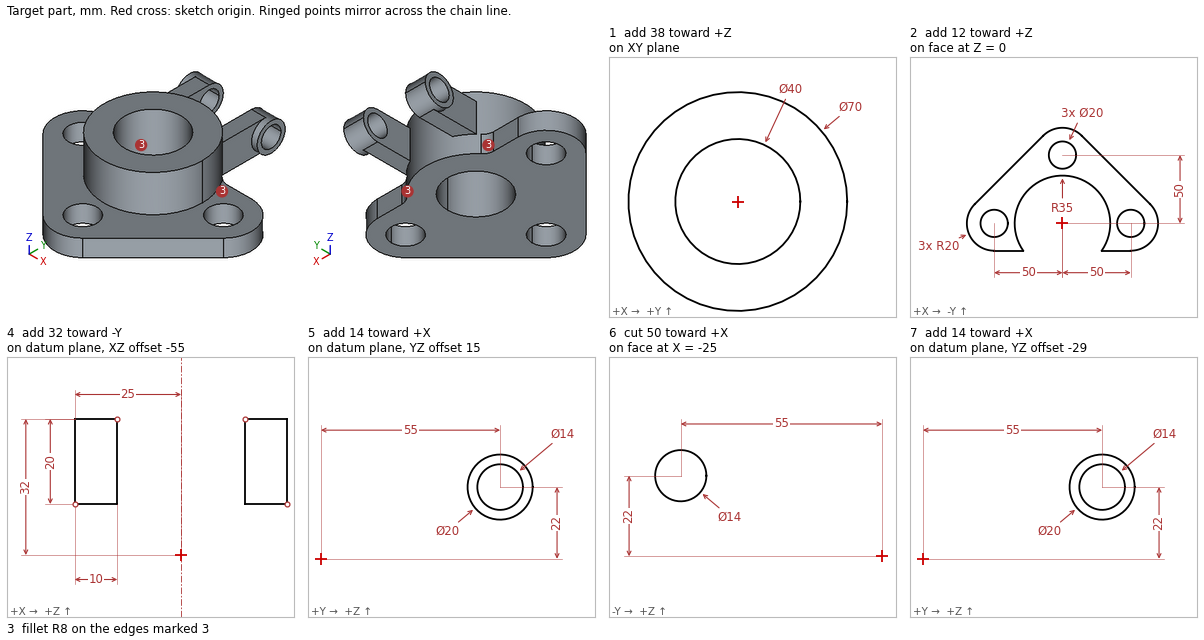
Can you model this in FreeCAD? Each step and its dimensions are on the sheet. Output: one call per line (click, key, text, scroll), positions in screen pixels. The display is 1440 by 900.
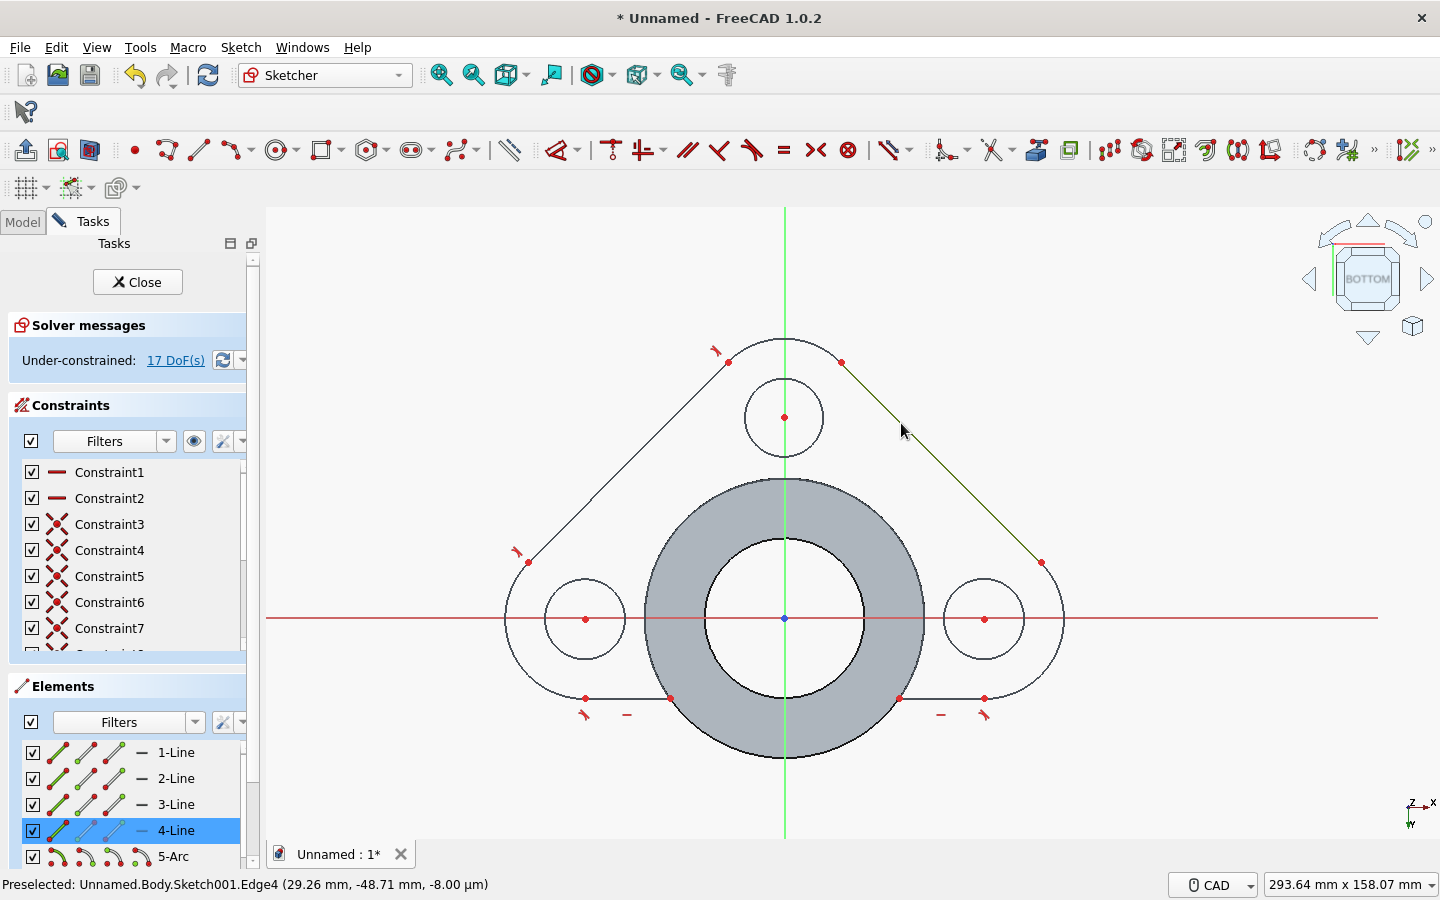
click(809, 343)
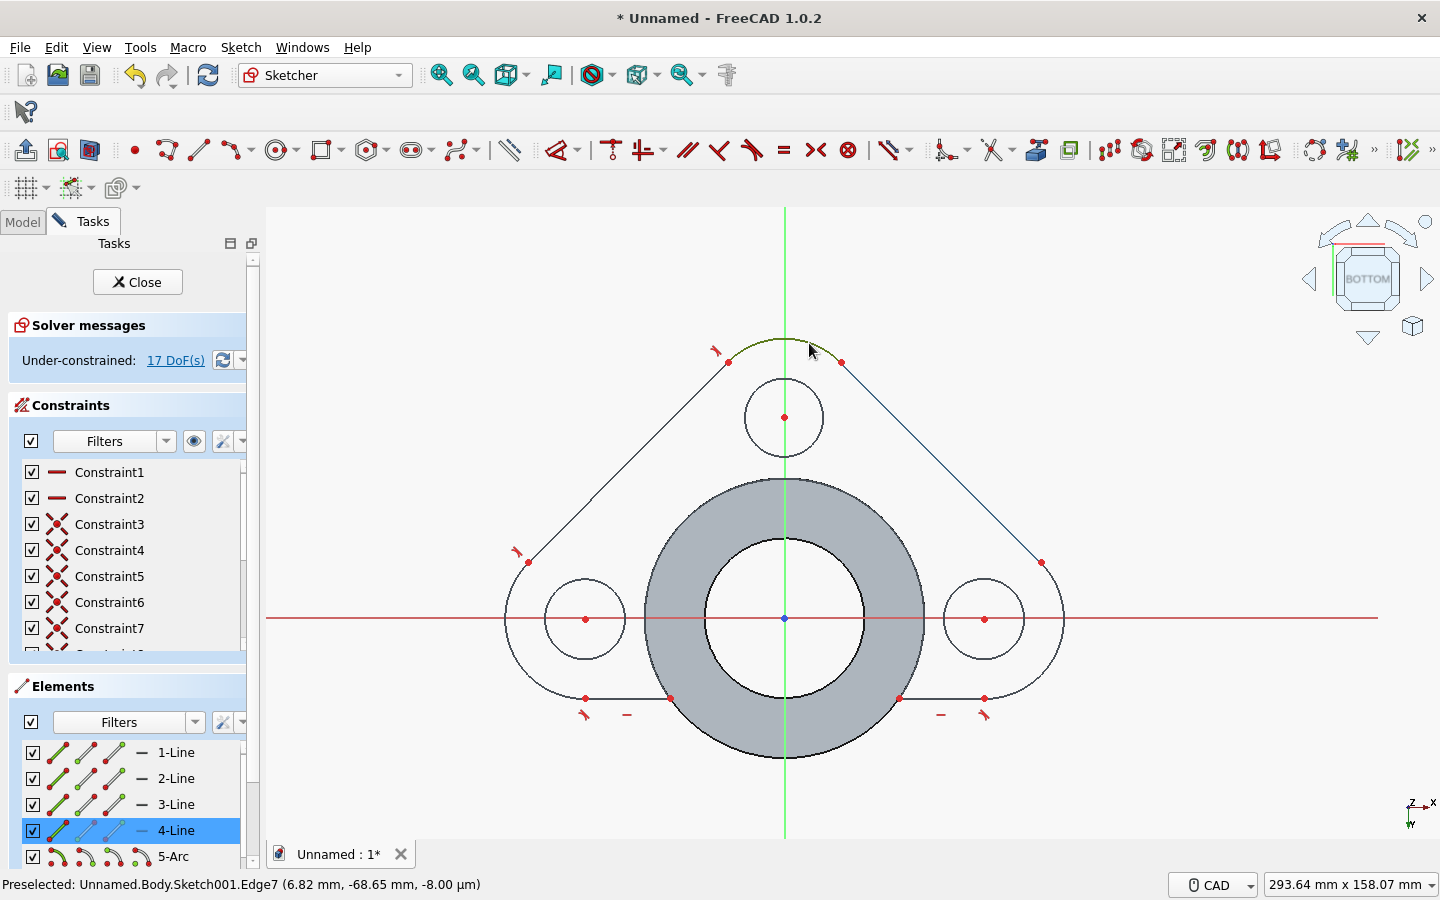
key(t)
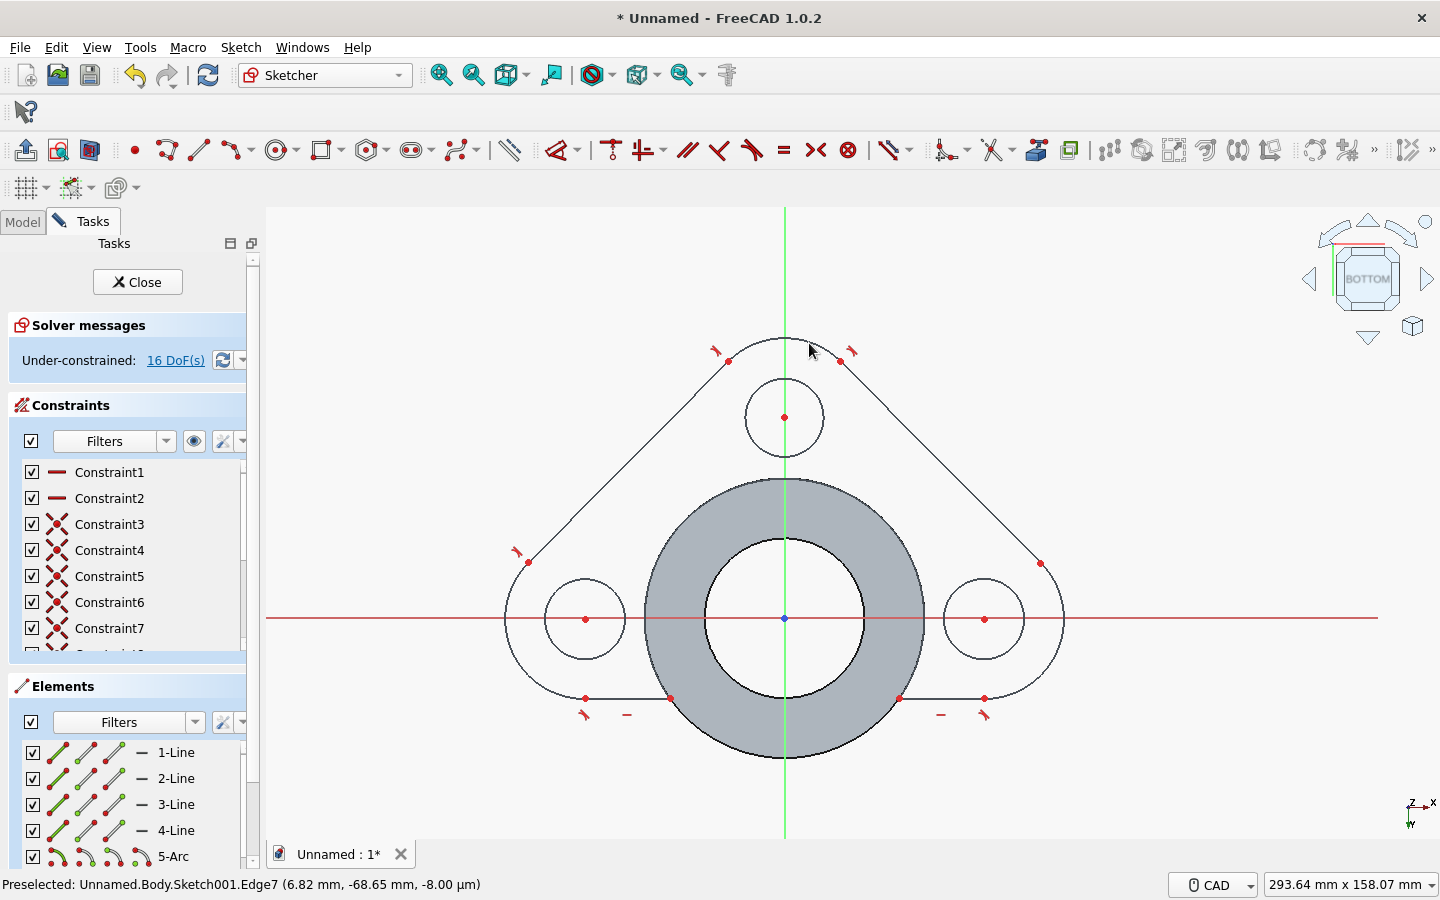
click(901, 422)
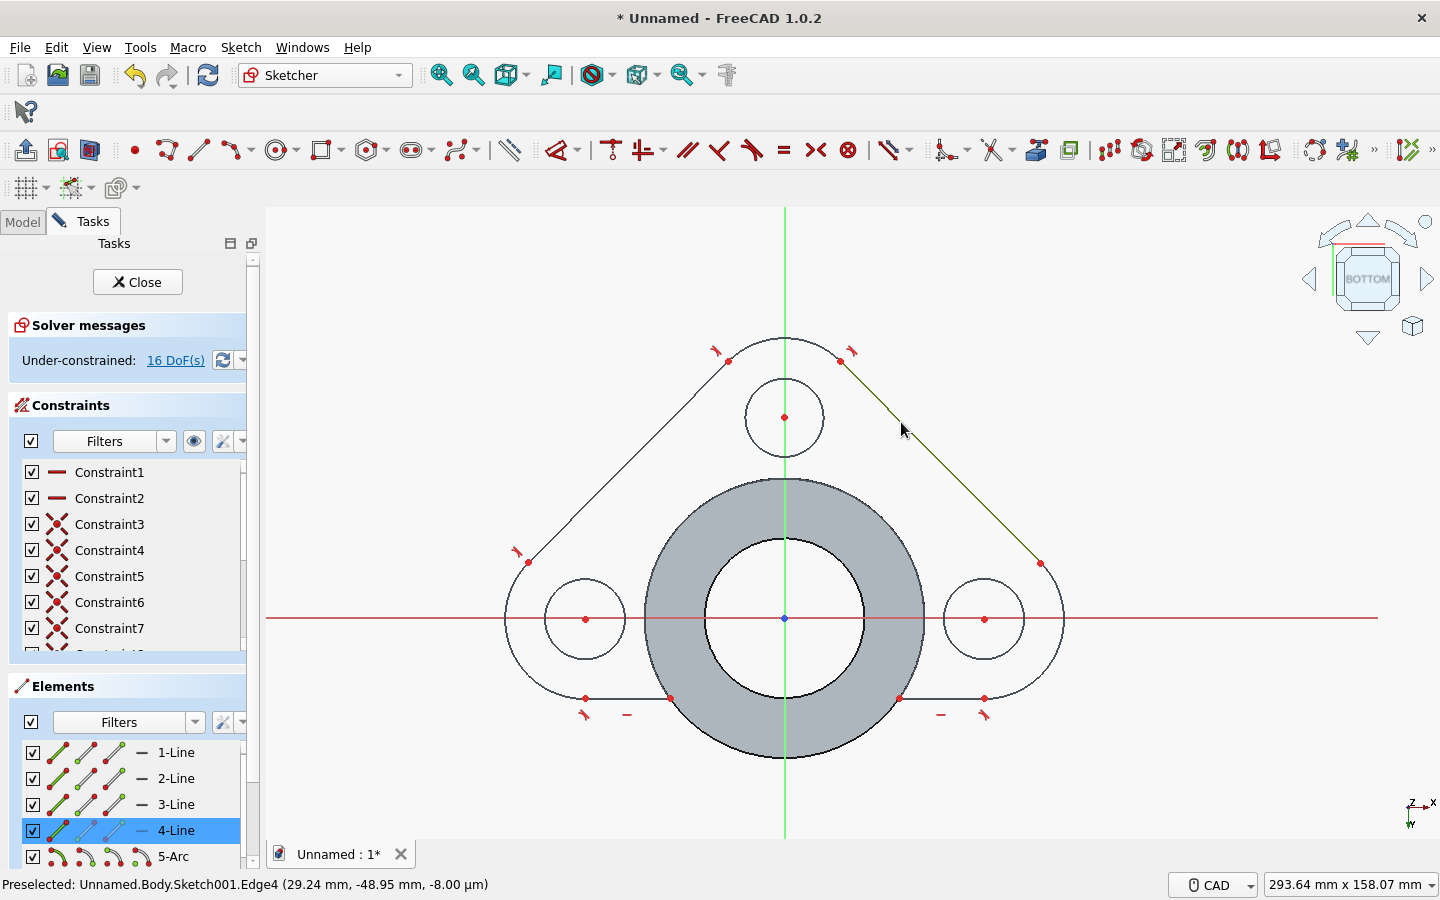
click(1036, 680)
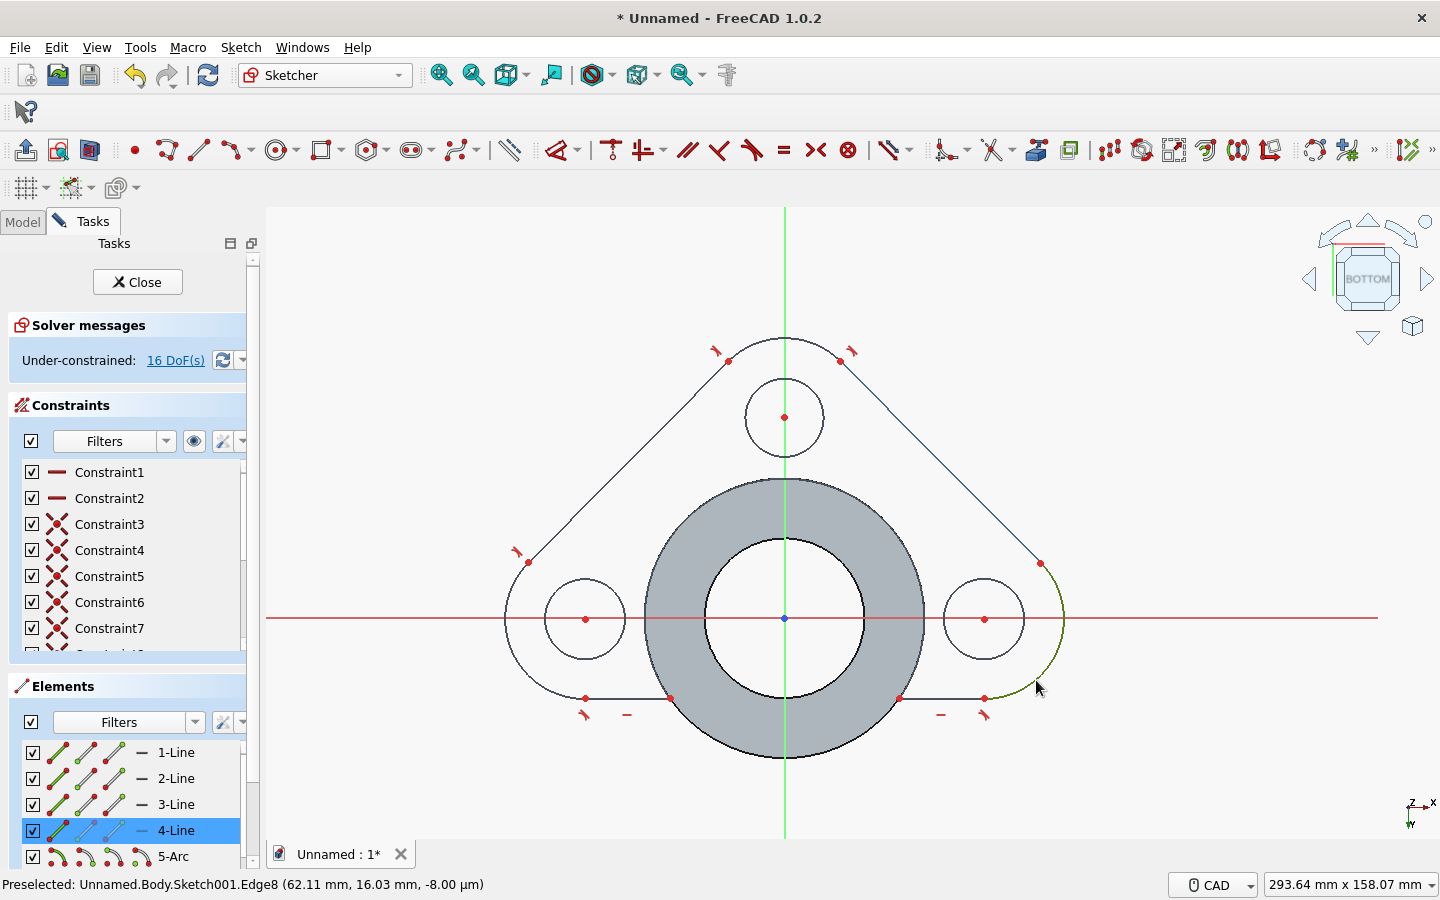
key(t)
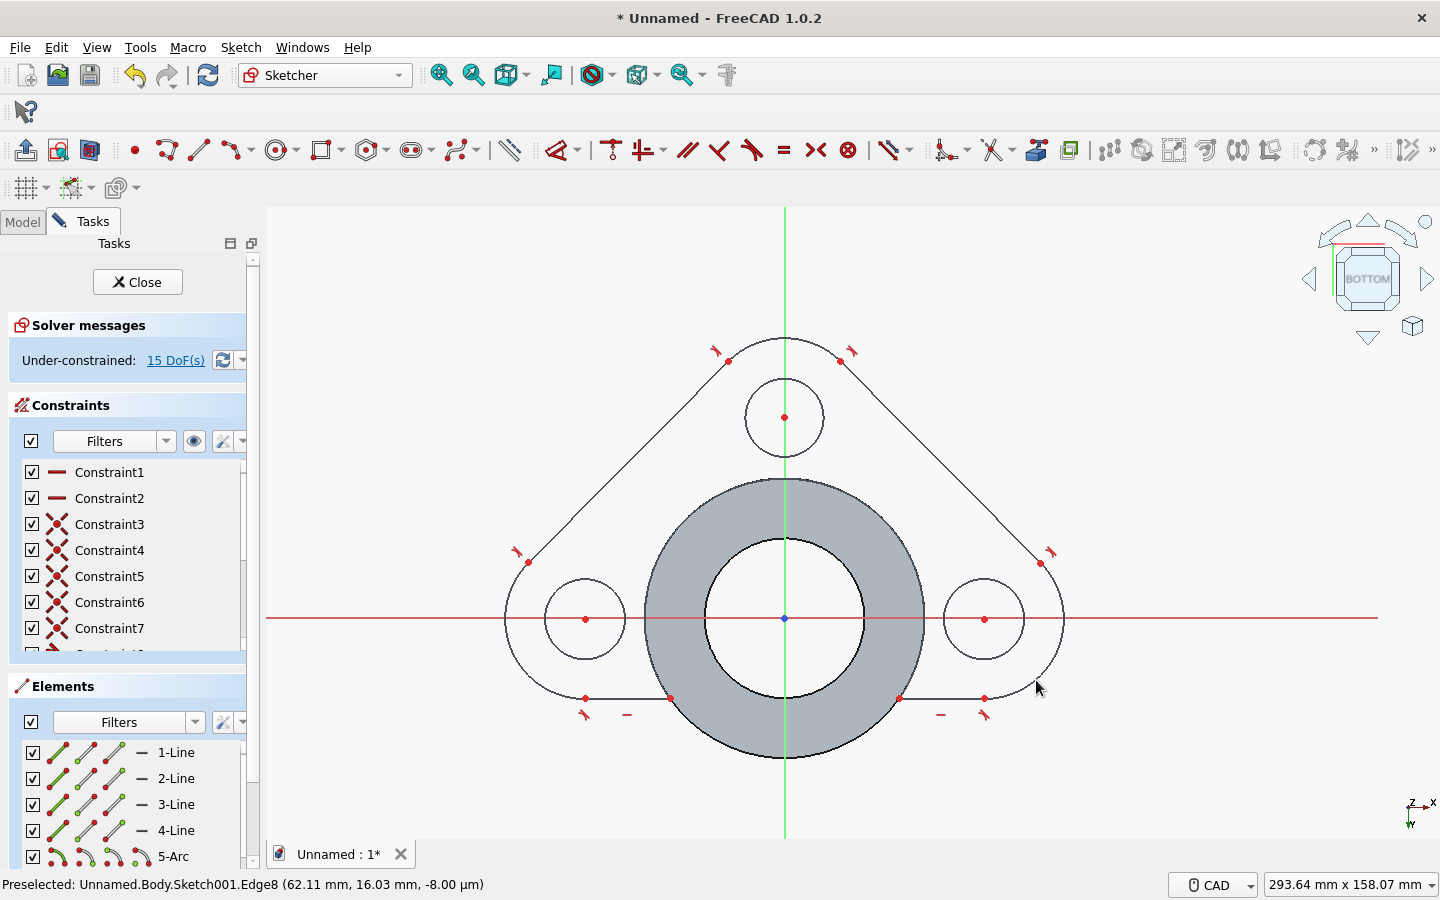
drag(775, 608, 795, 629)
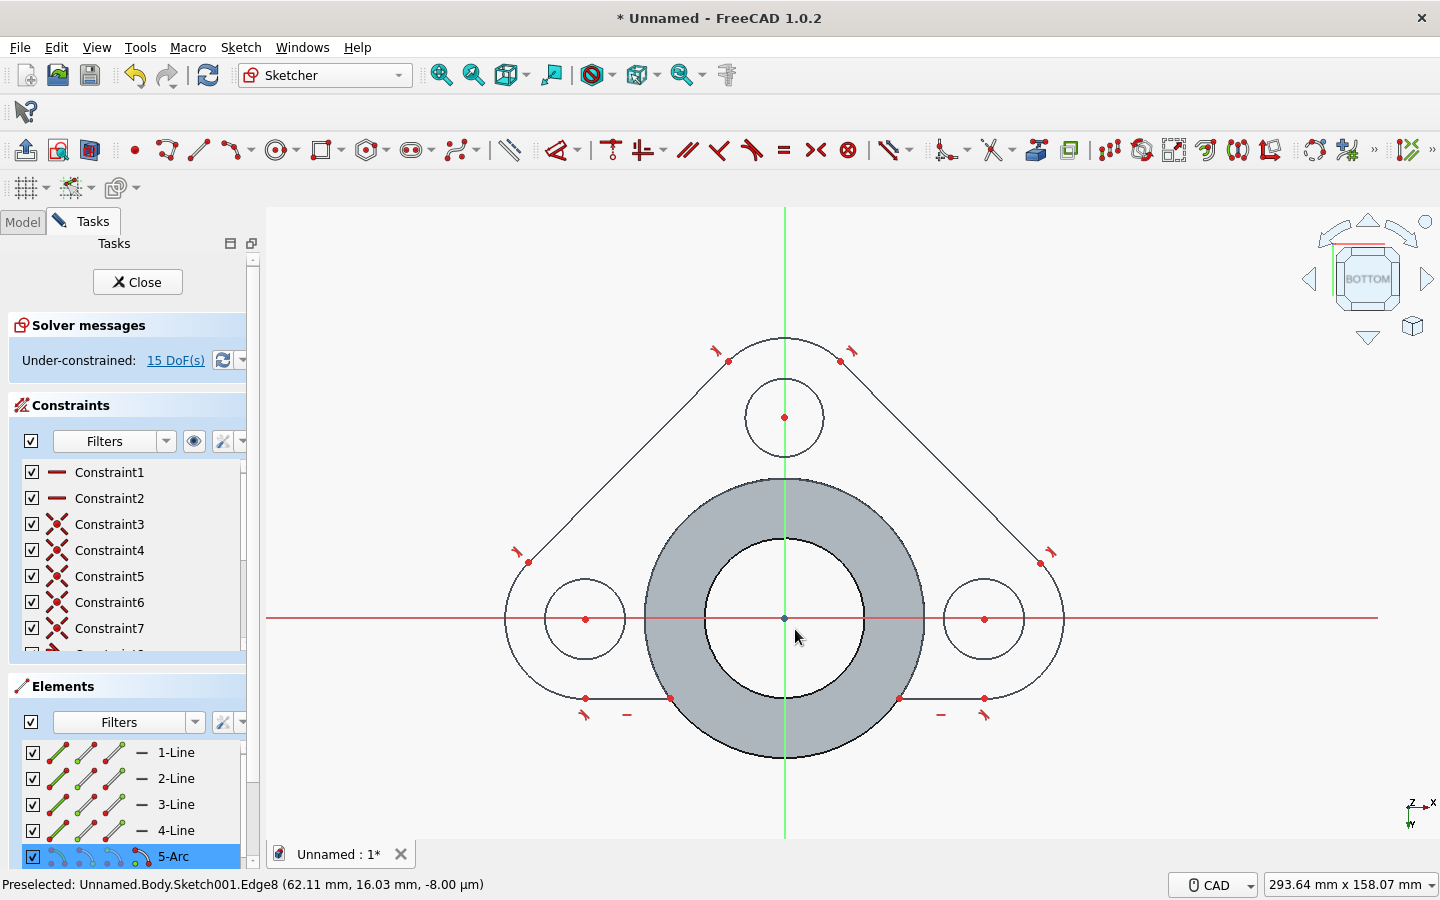
key(c)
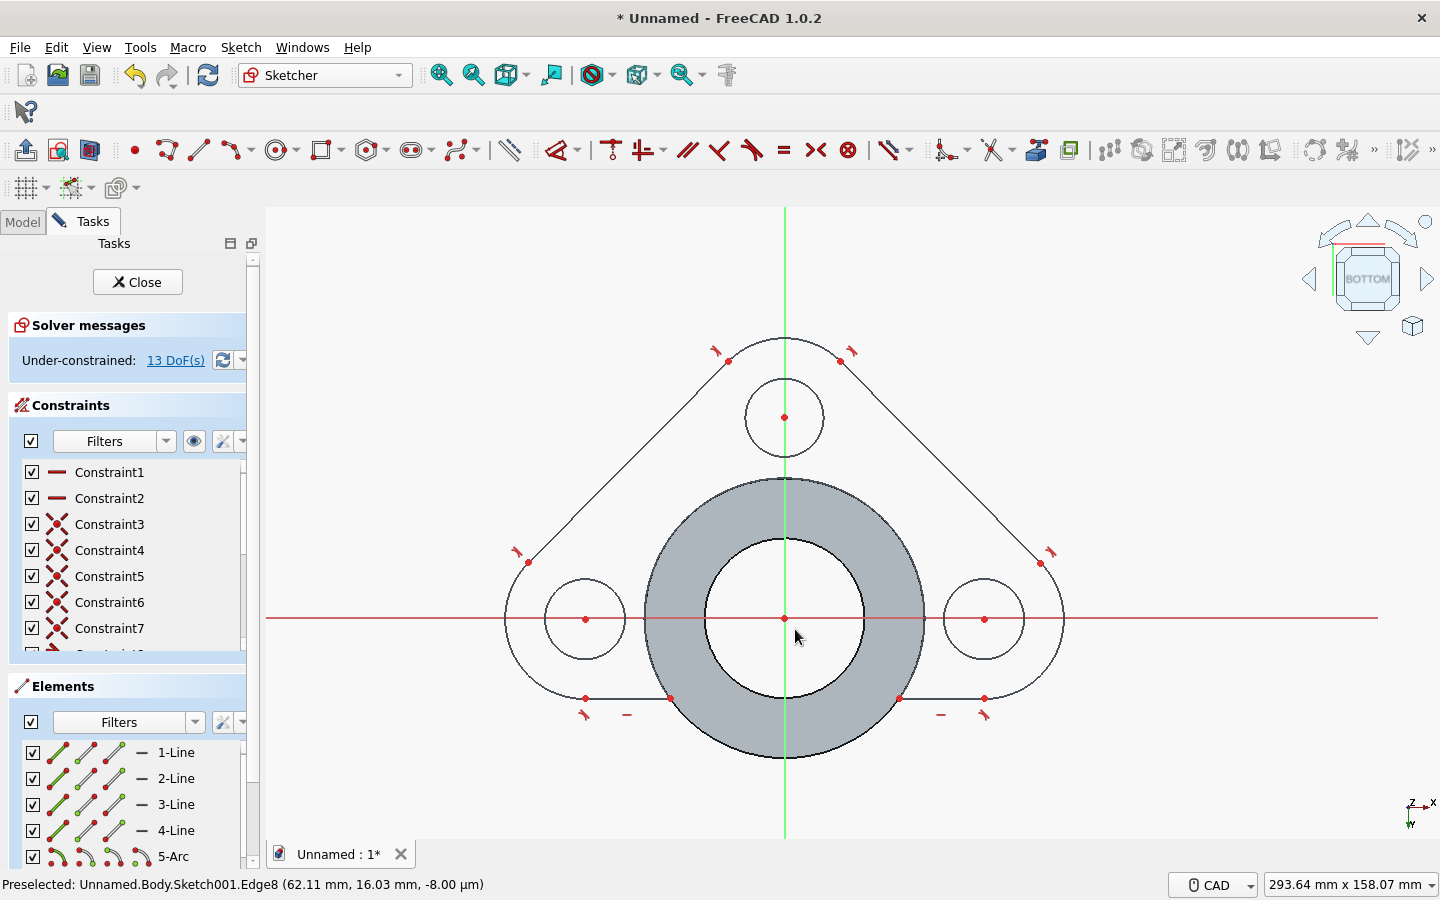
click(533, 680)